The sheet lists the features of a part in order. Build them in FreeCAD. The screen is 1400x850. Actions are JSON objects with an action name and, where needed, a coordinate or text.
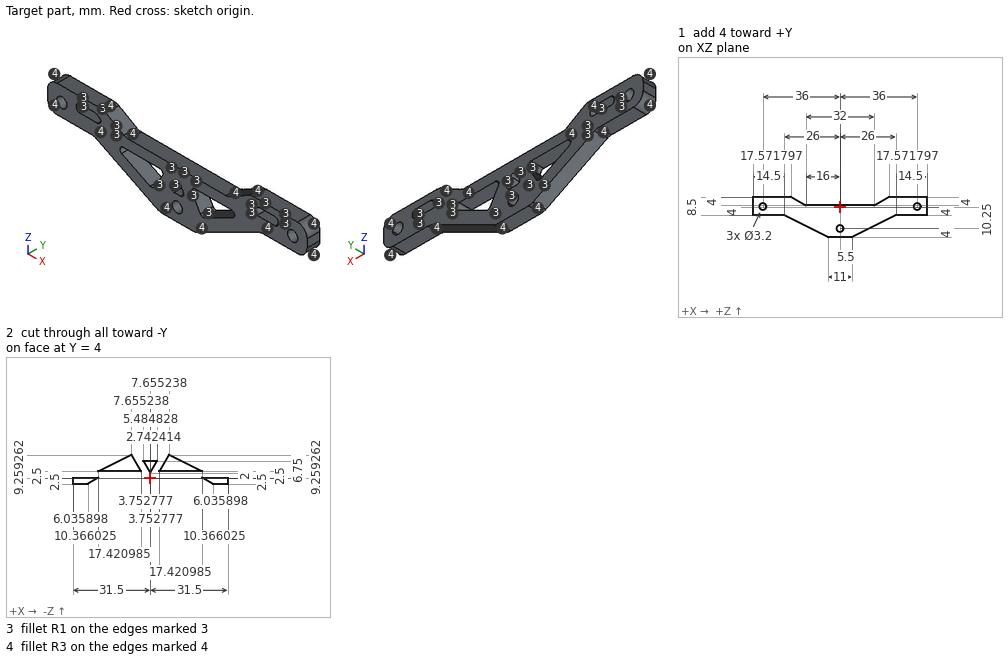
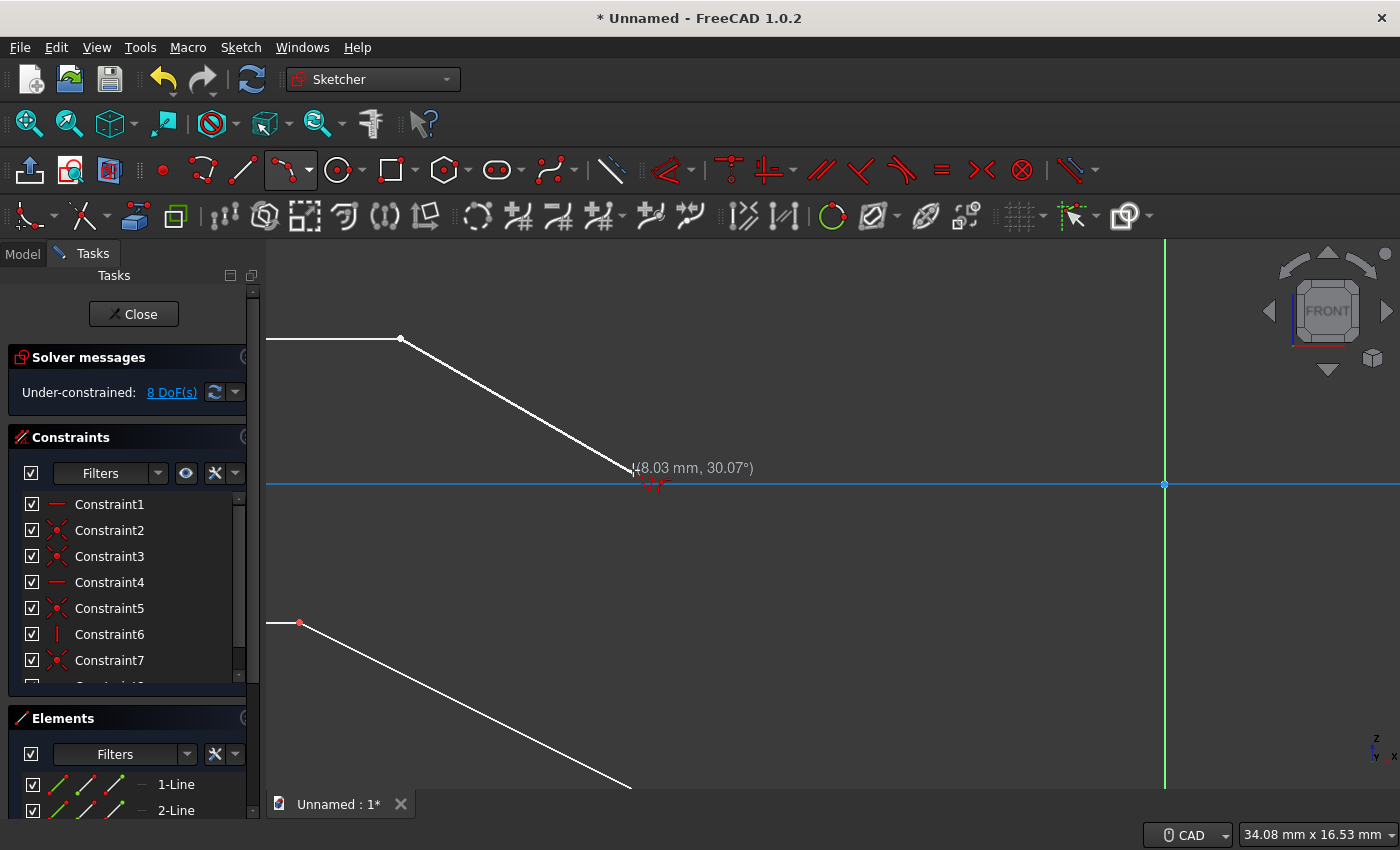
{"action": "left_click", "coordinate": [632, 468]}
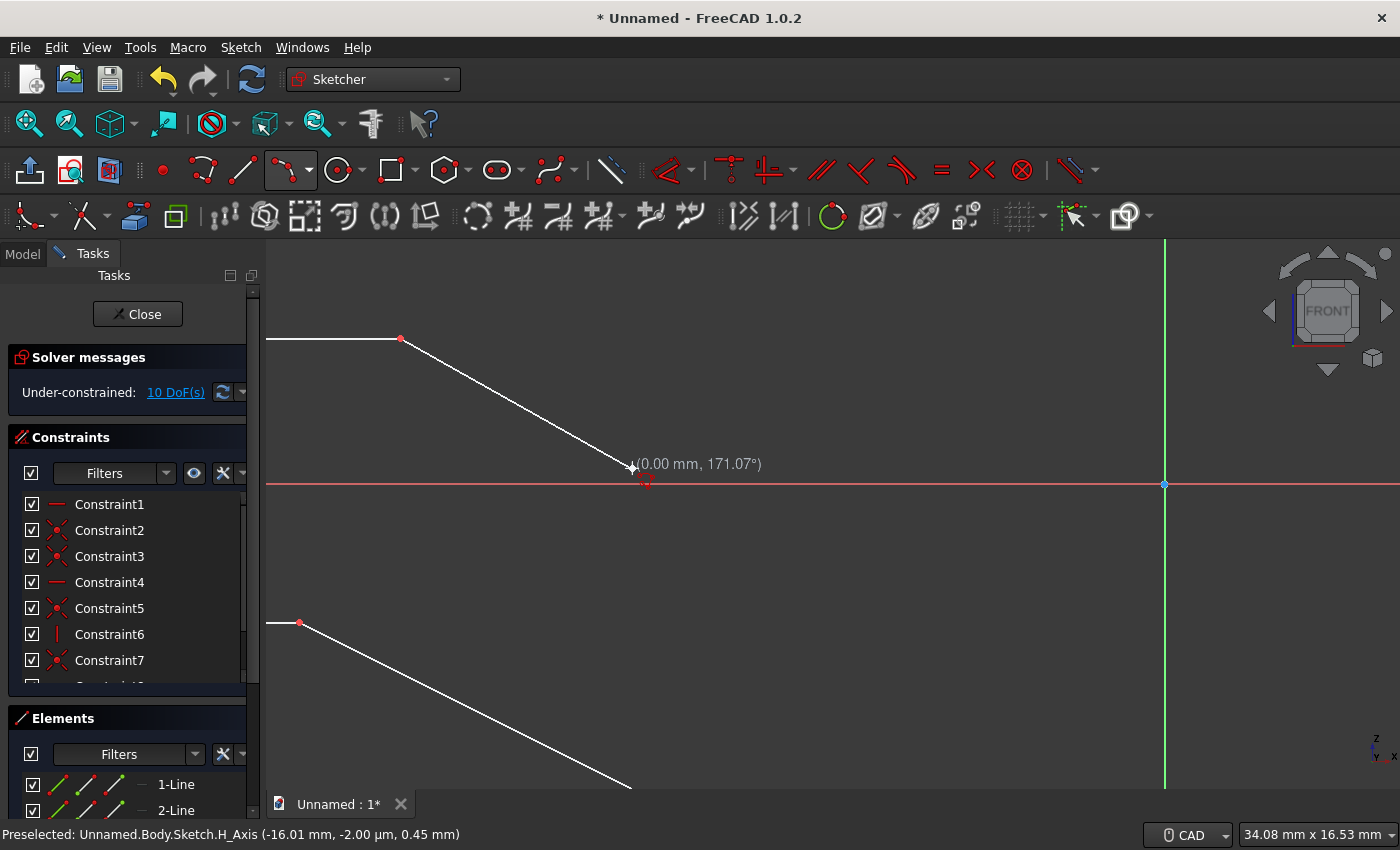
{"action": "scroll", "coordinate": [634, 471], "scroll_direction": "down", "scroll_amount": 7}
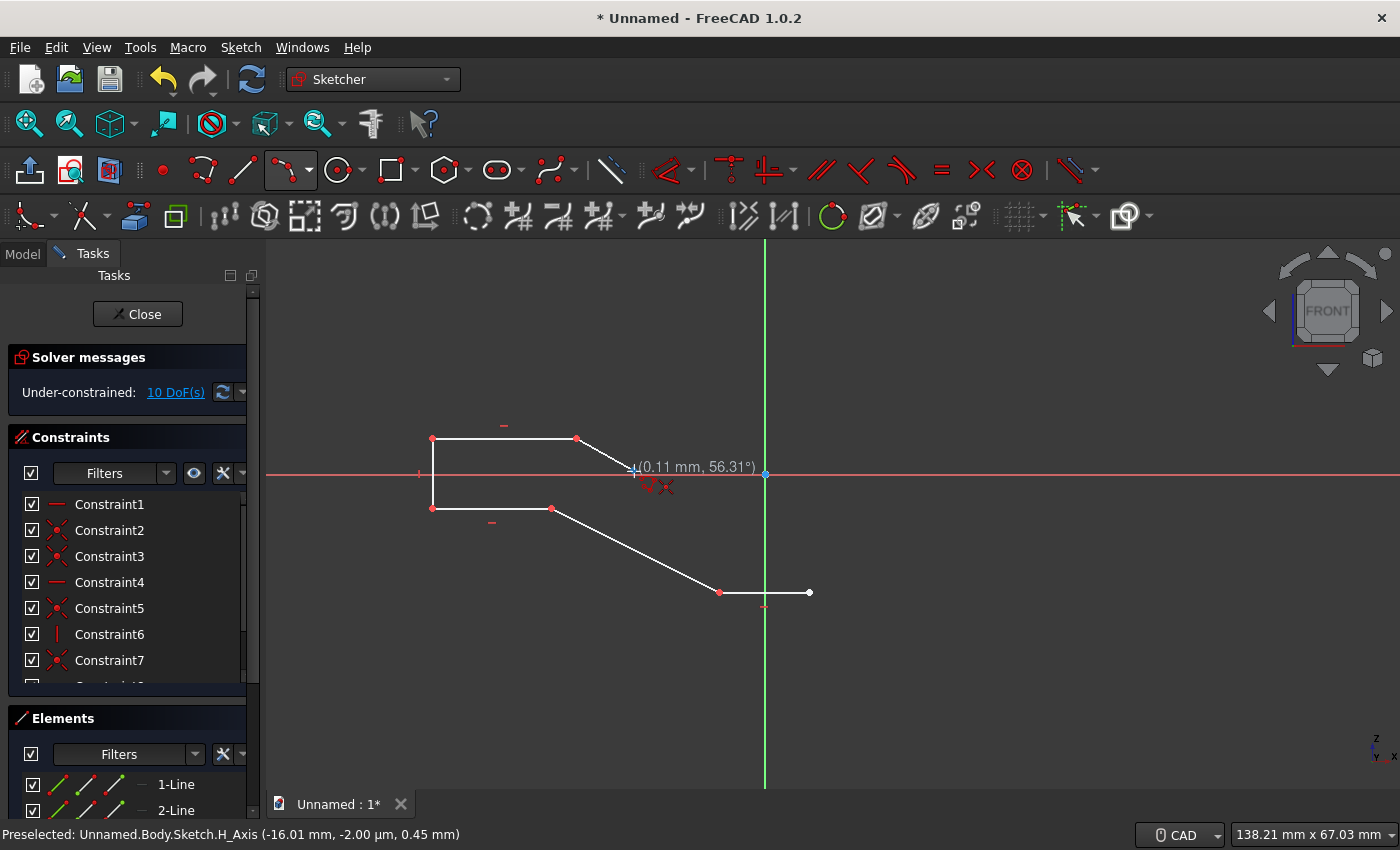
{"action": "scroll", "coordinate": [896, 470], "scroll_direction": "up", "scroll_amount": 7}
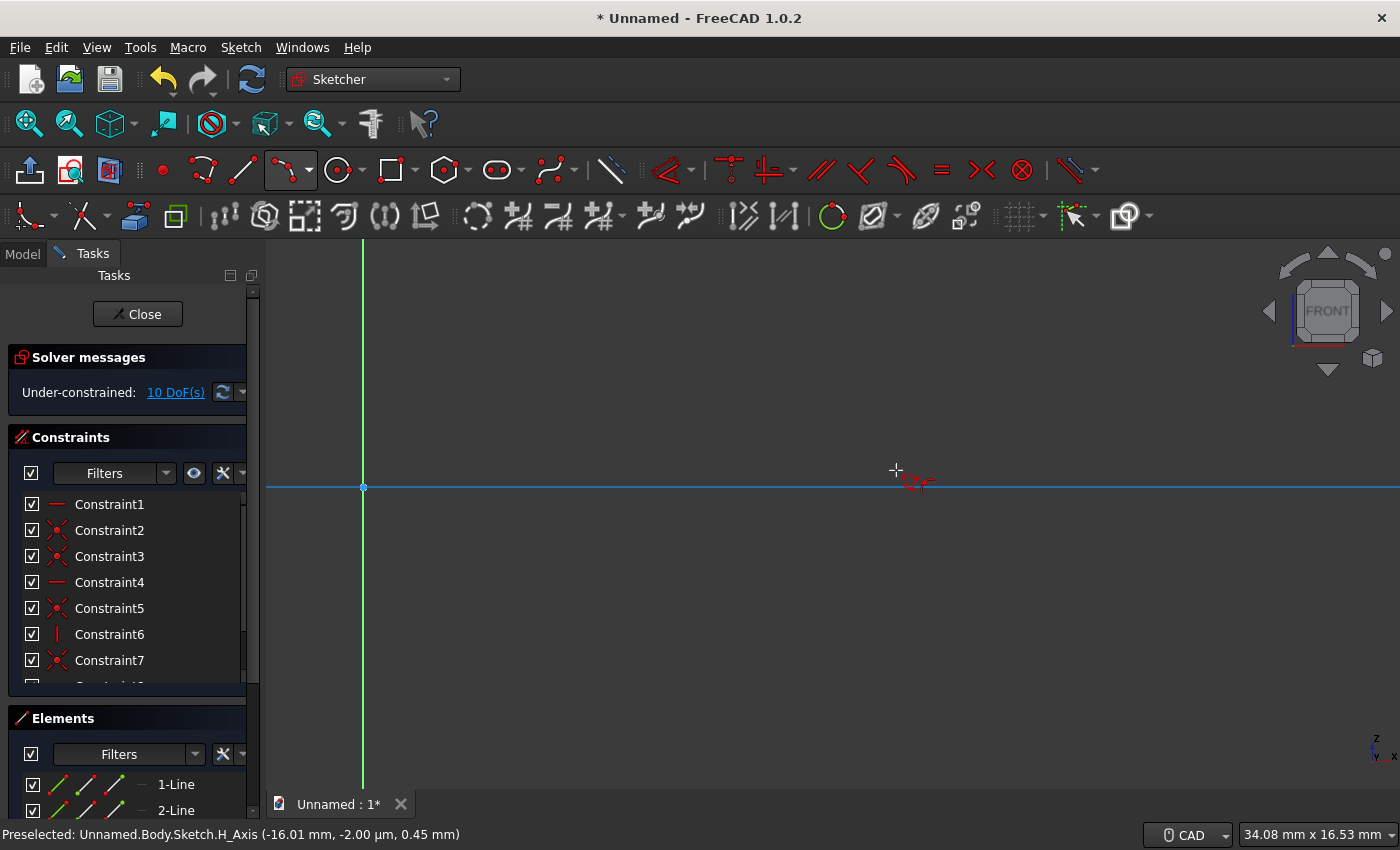
{"action": "left_click", "coordinate": [896, 471]}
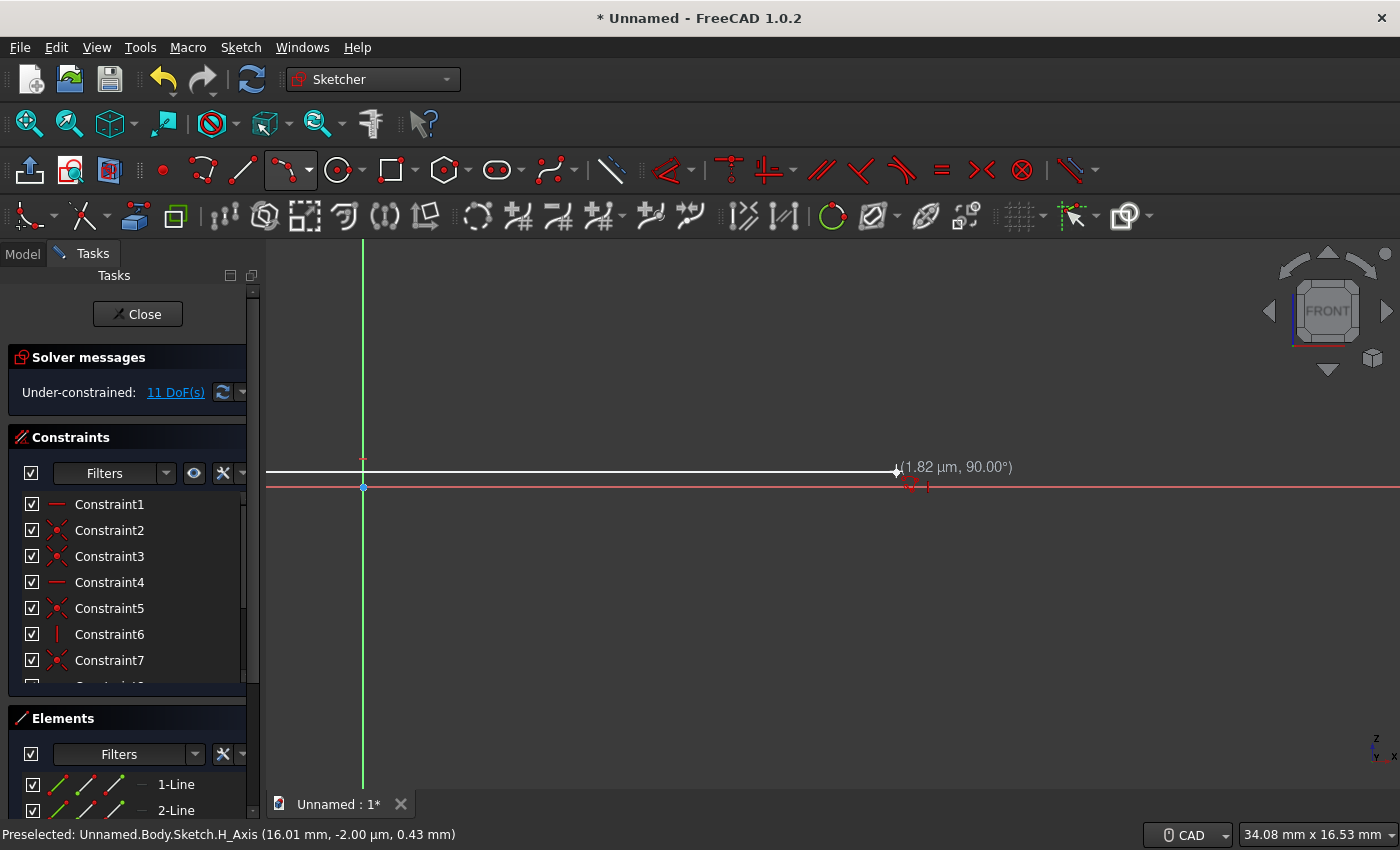
{"action": "scroll", "coordinate": [896, 470], "scroll_direction": "down", "scroll_amount": 7}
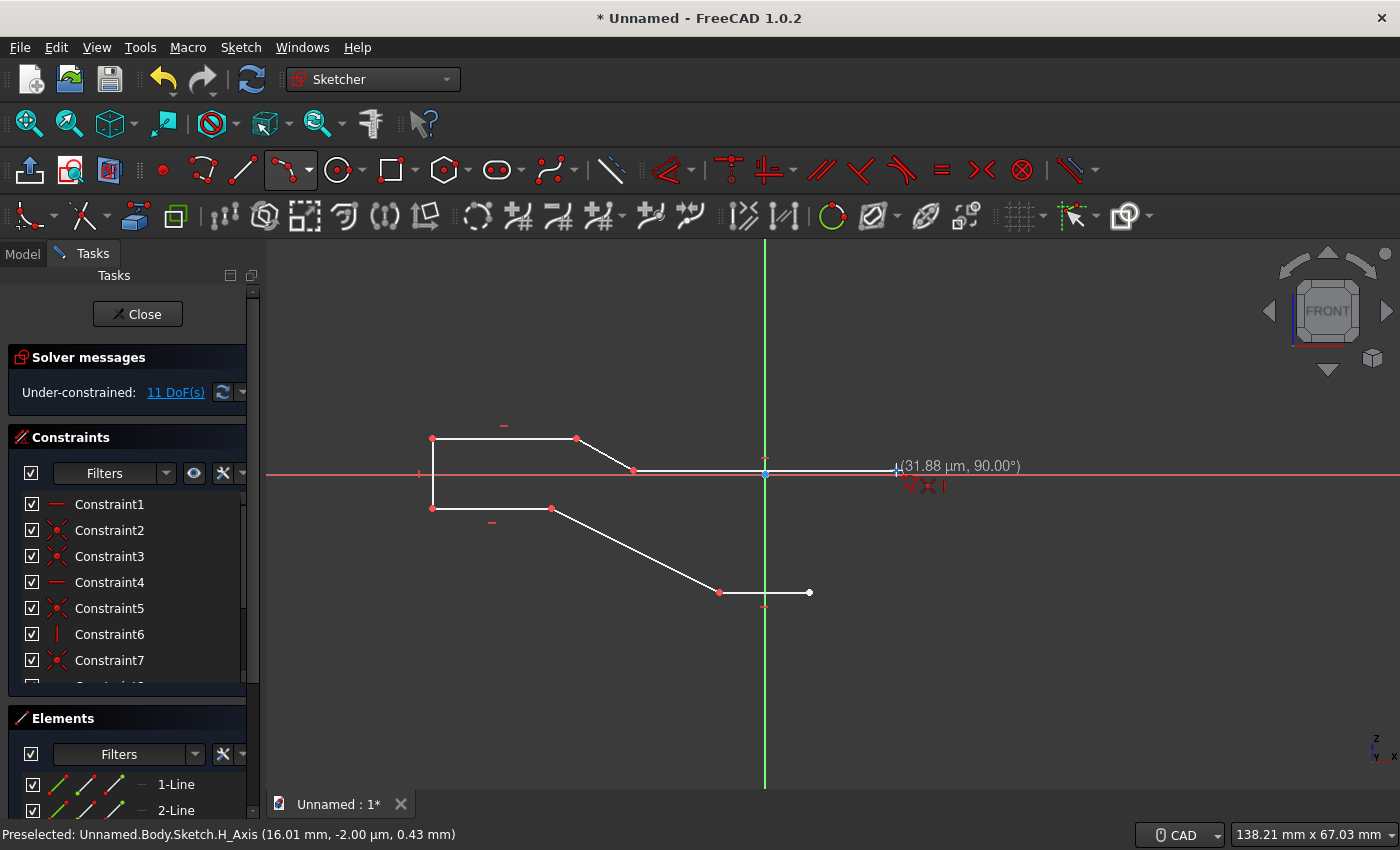
{"action": "left_click", "coordinate": [953, 438]}
{"action": "left_click", "coordinate": [1097, 438]}
{"action": "left_click", "coordinate": [1097, 507]}
{"action": "left_click", "coordinate": [978, 507]}
{"action": "left_click", "coordinate": [810, 593]}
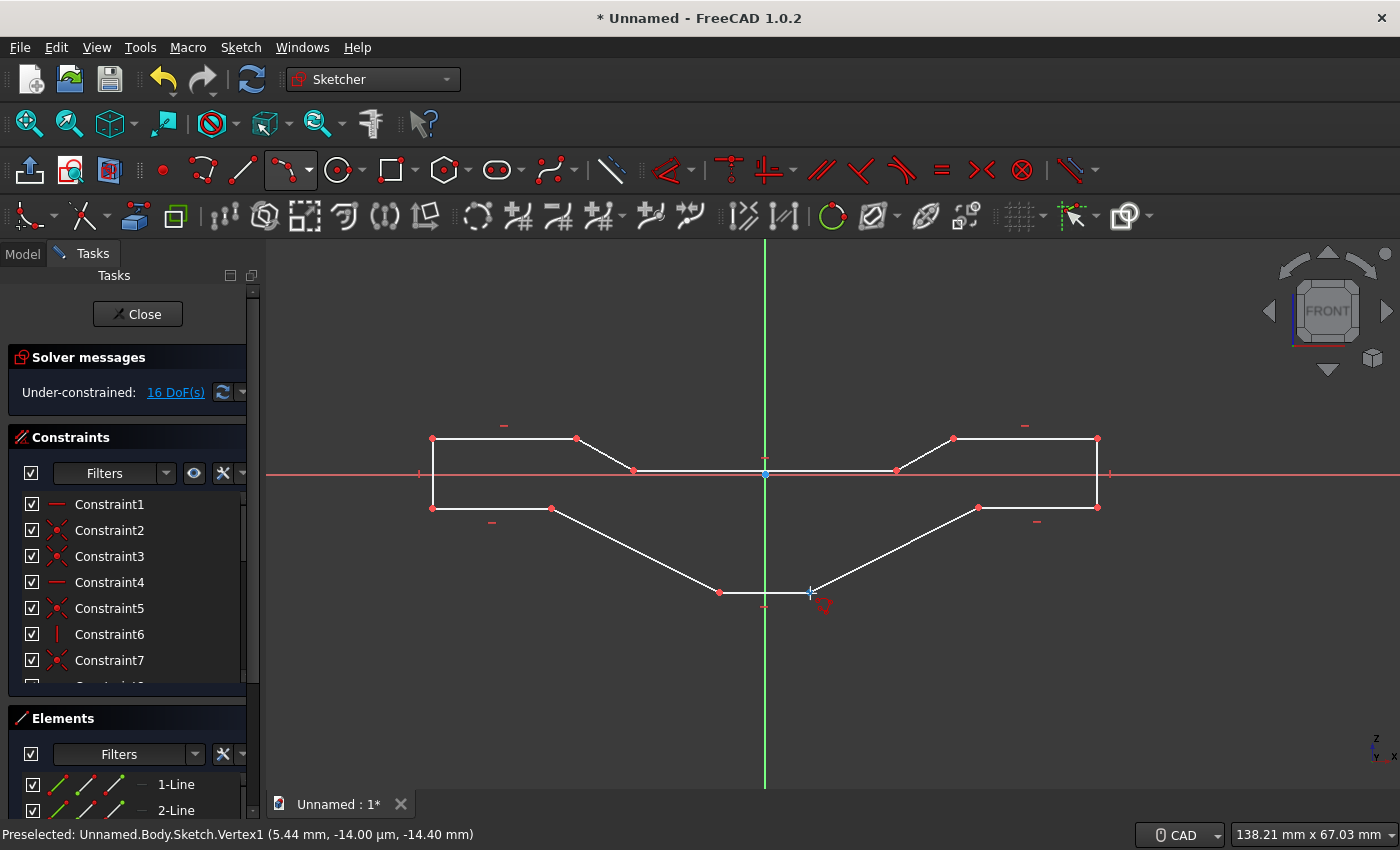
{"action": "left_click", "coordinate": [338, 170]}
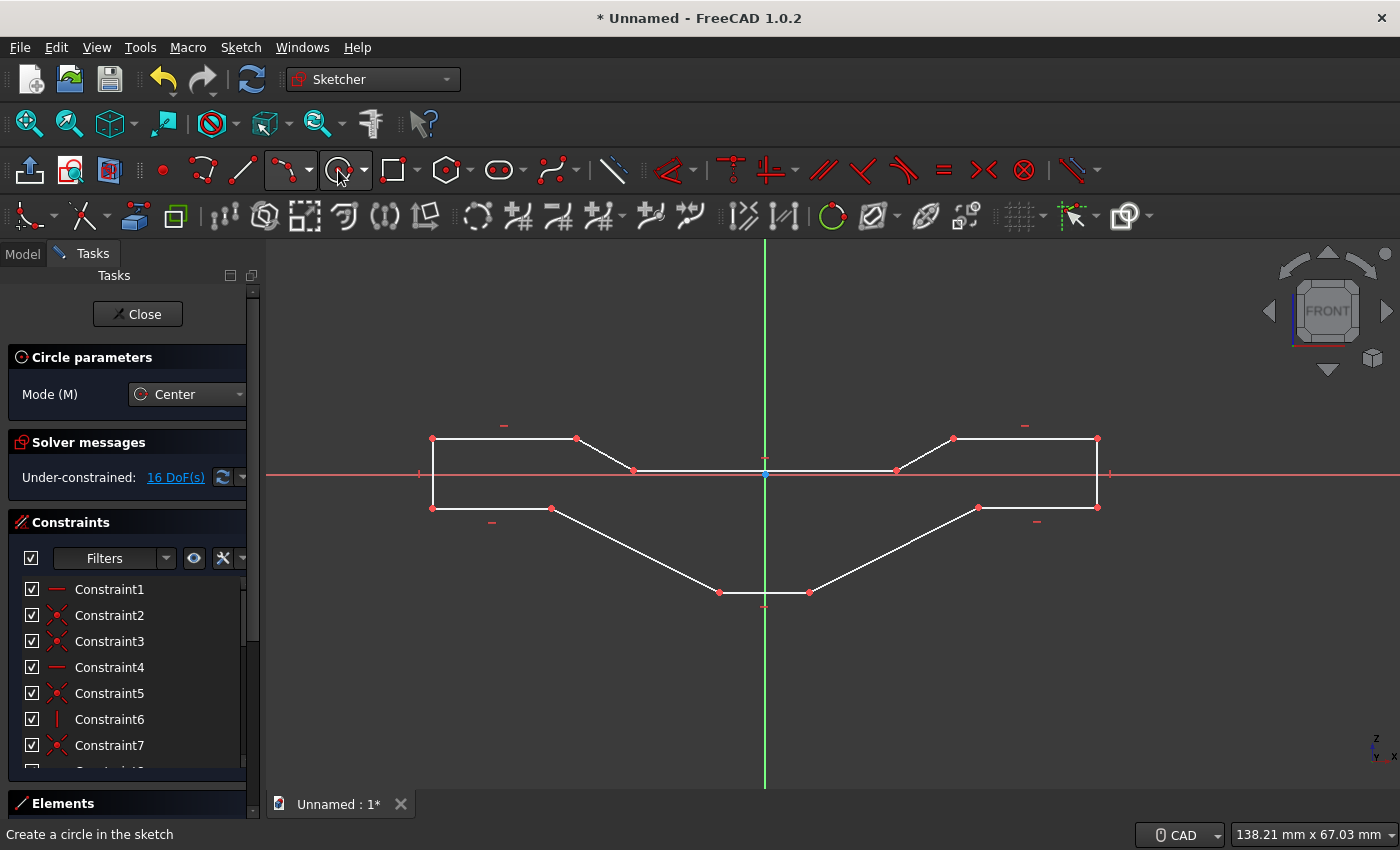
{"action": "scroll", "coordinate": [470, 475], "scroll_direction": "up", "scroll_amount": 3}